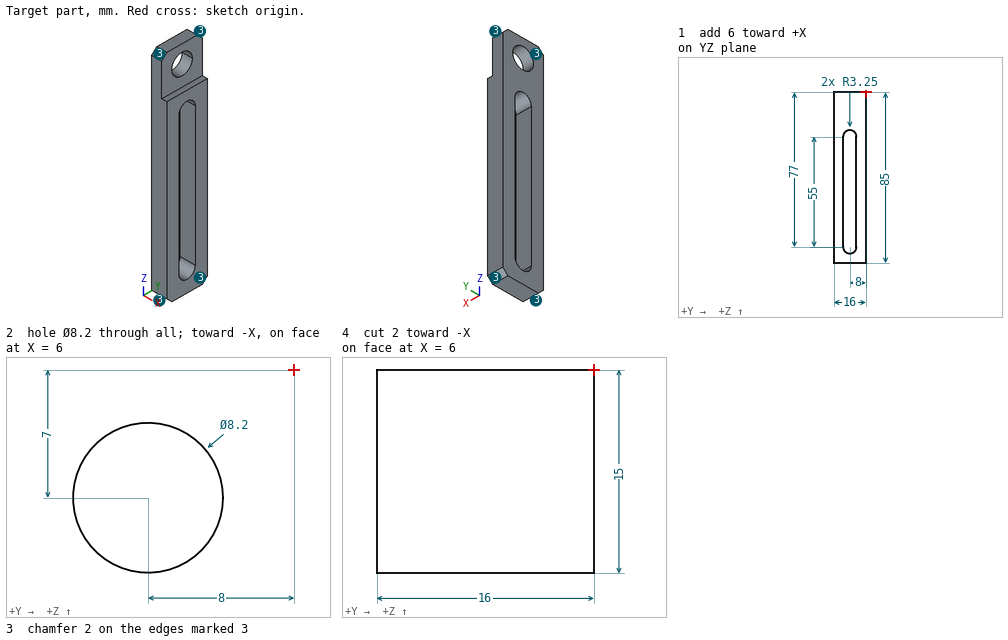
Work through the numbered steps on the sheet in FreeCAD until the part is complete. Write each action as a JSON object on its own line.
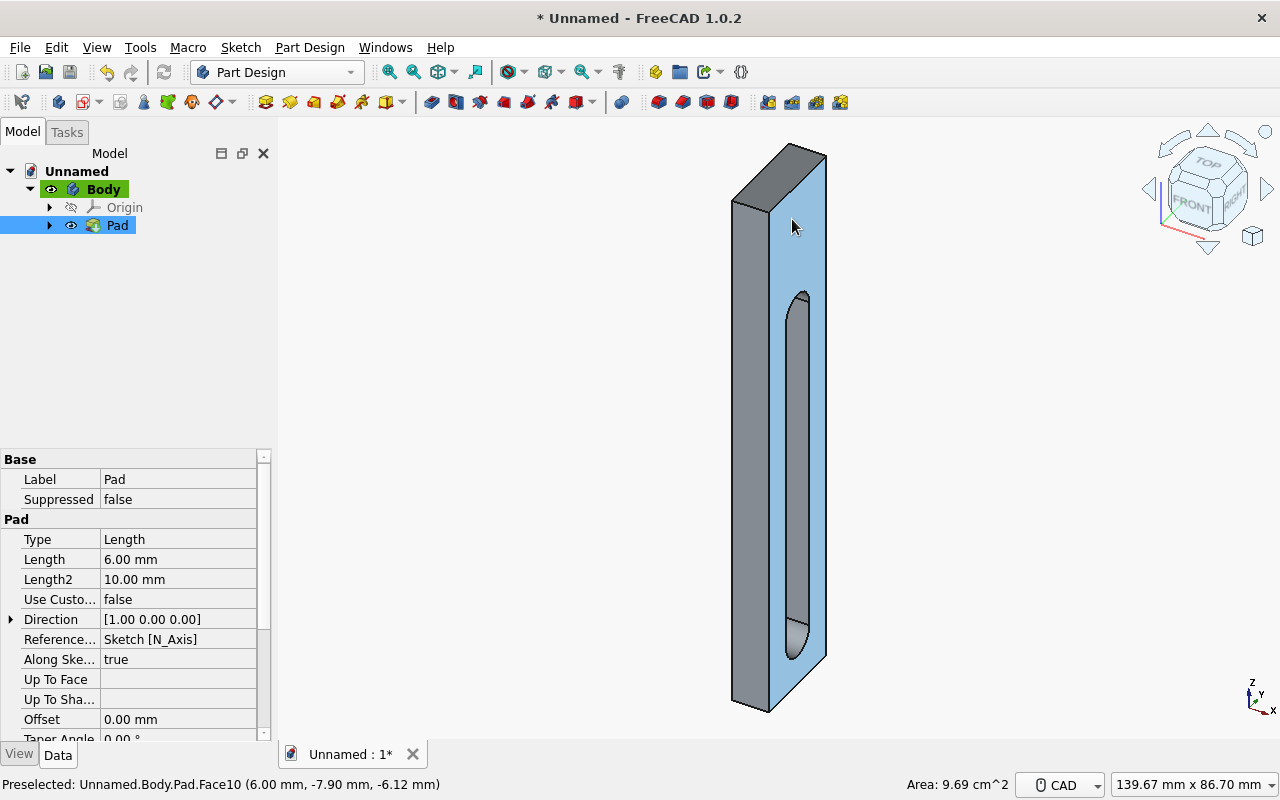
{"action": "left_click", "coordinate": [84, 102]}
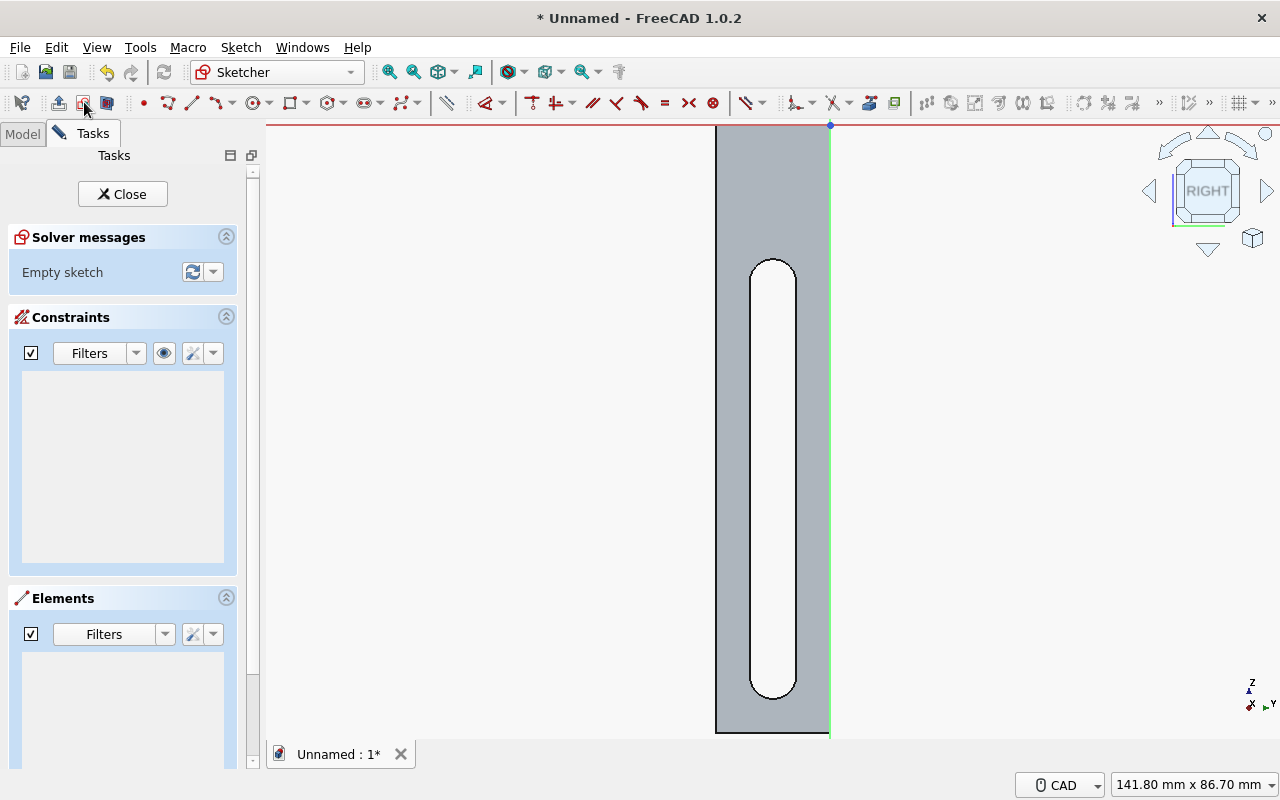
{"action": "scroll", "coordinate": [704, 429], "scroll_direction": "down", "scroll_amount": 5}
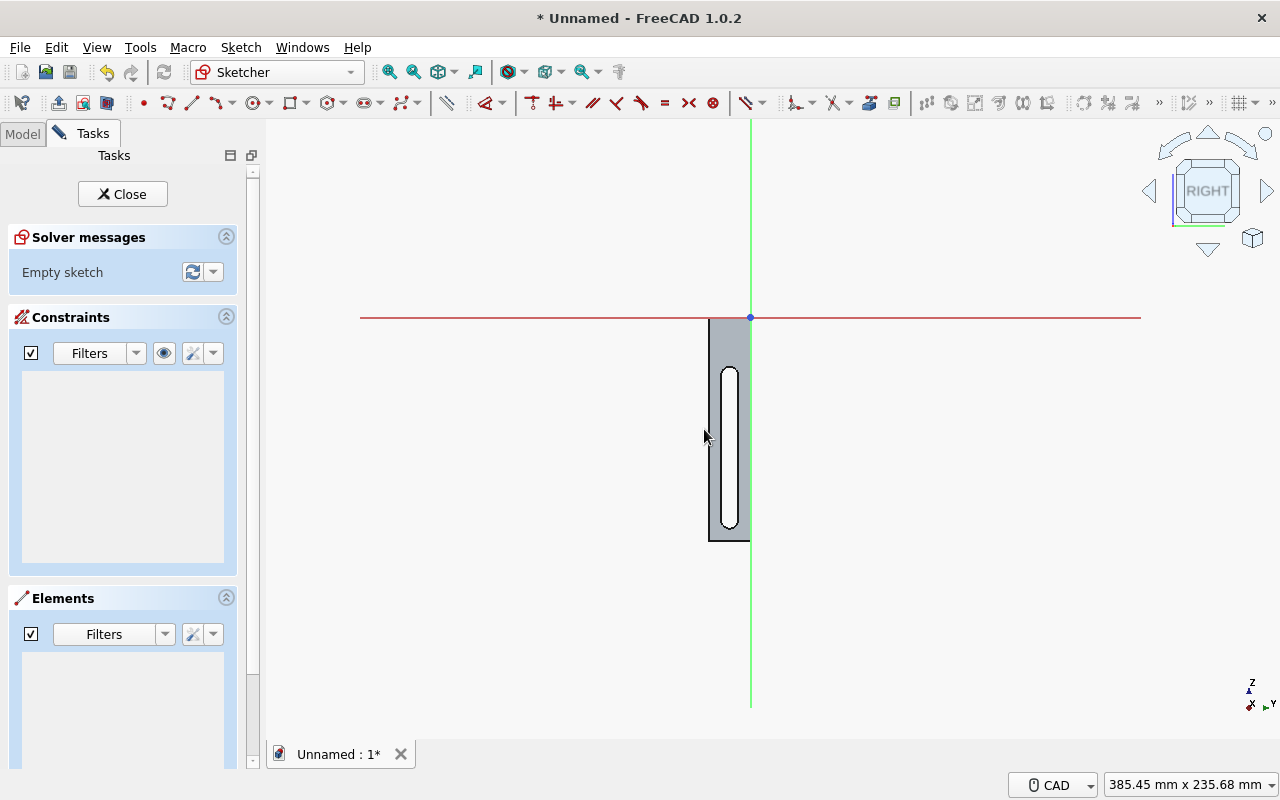
{"action": "scroll", "coordinate": [737, 324], "scroll_direction": "up", "scroll_amount": 13}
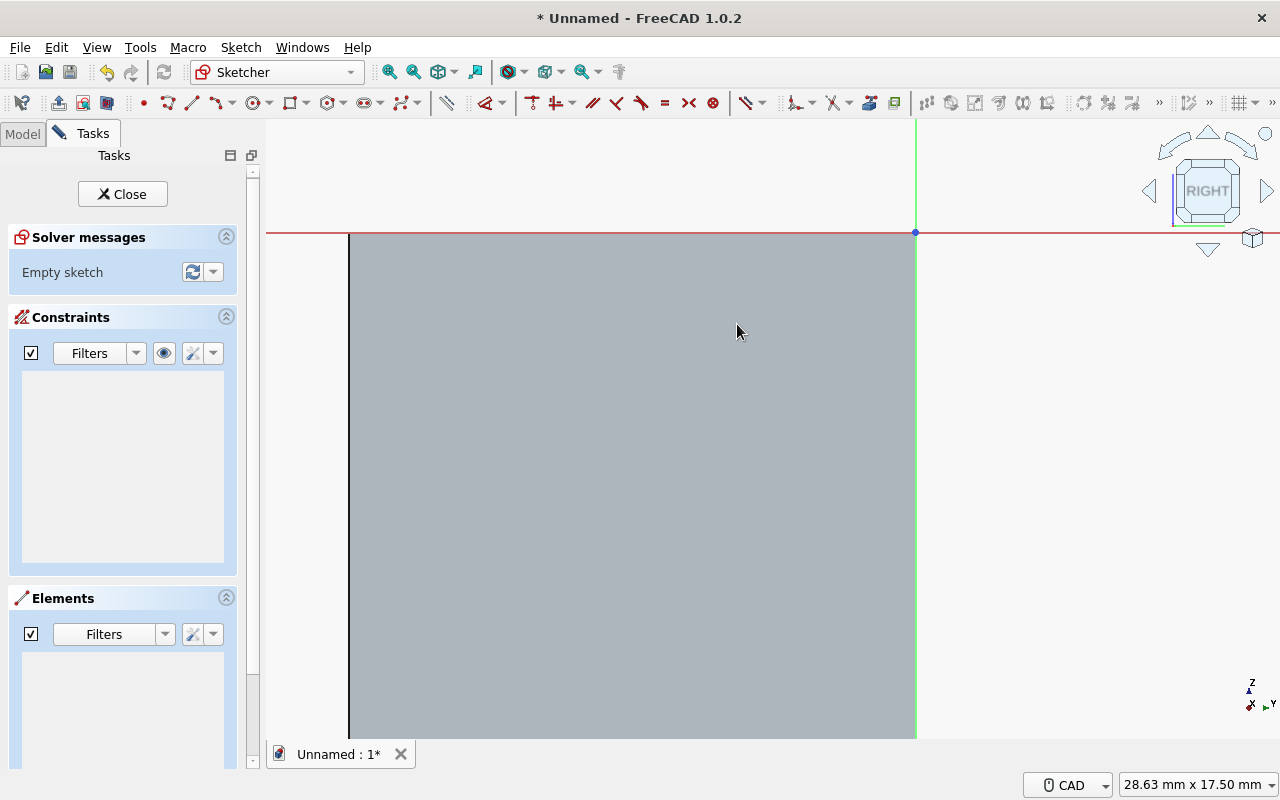
{"action": "key", "text": "g c"}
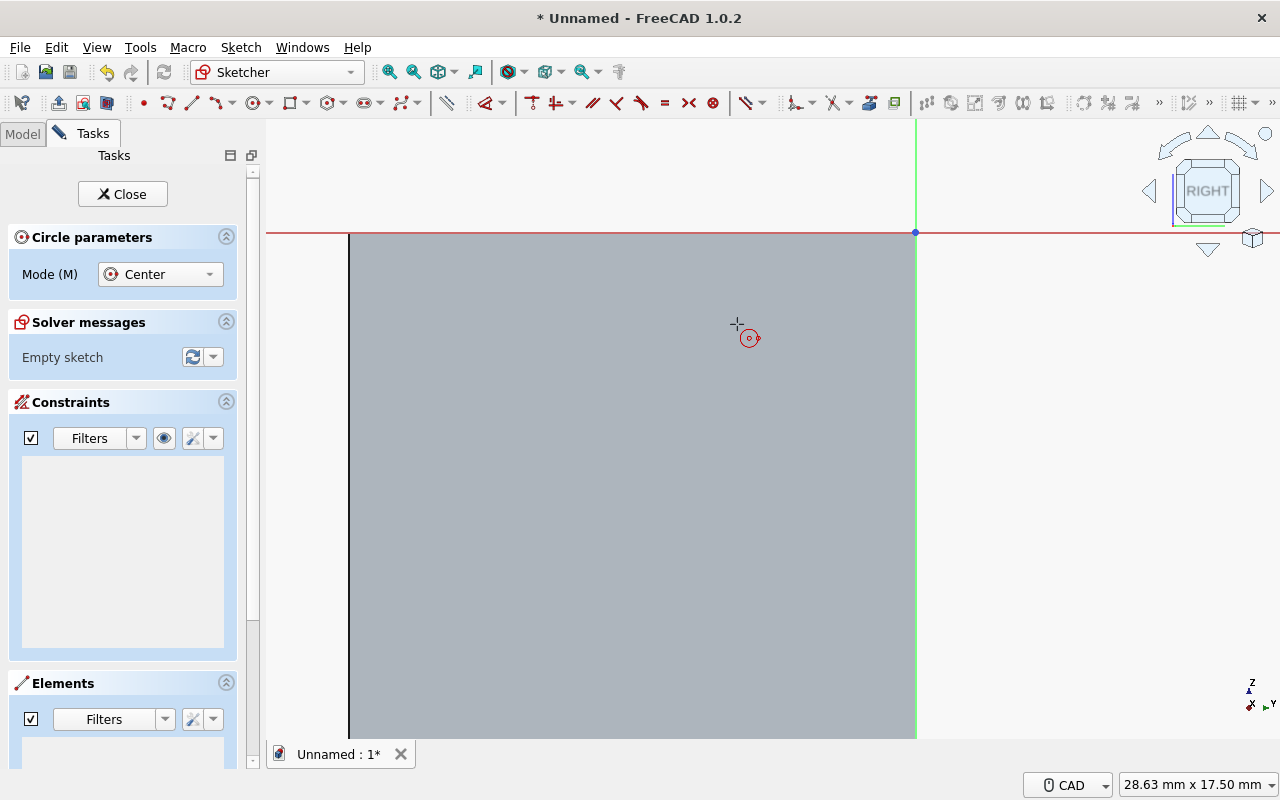
{"action": "left_click", "coordinate": [632, 480]}
{"action": "mouse_move", "coordinate": [735, 378]}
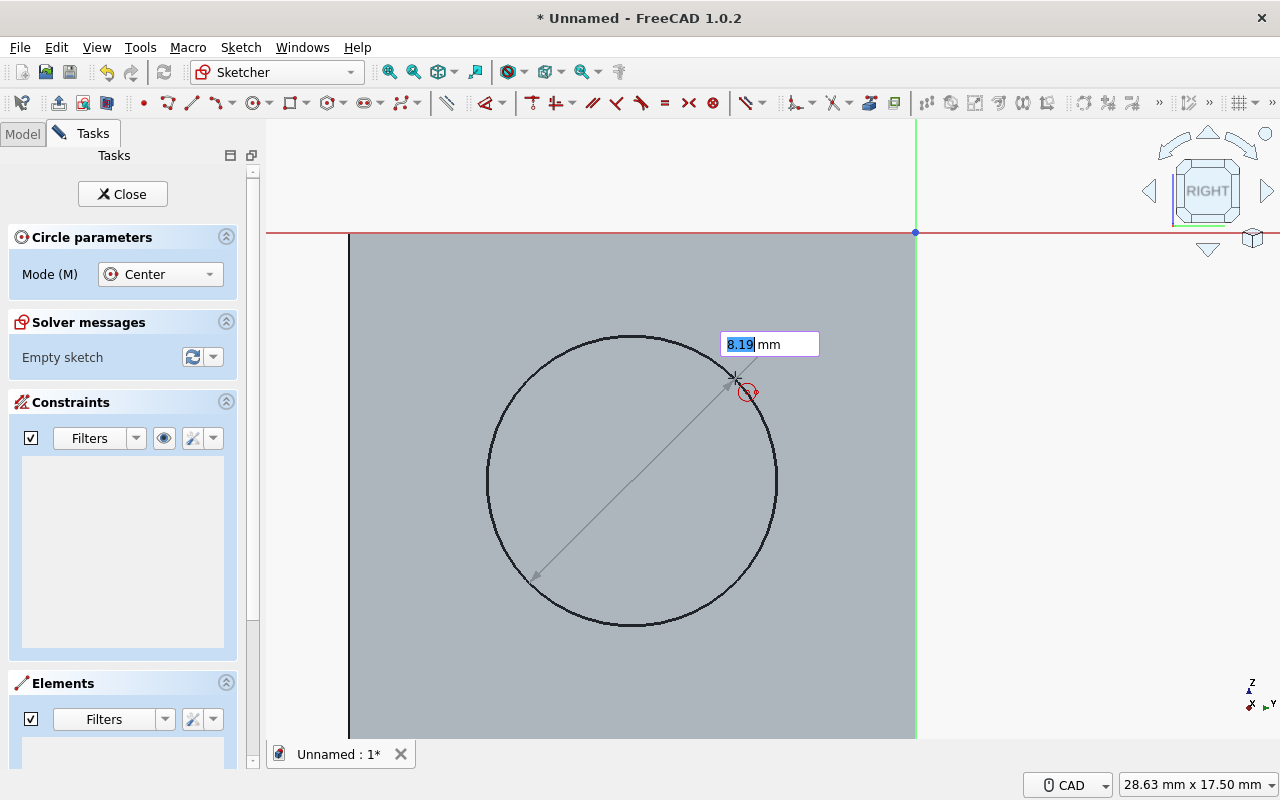
{"action": "type", "text": "8.2"}
{"action": "key", "text": "Return"}
{"action": "key", "text": "Escape"}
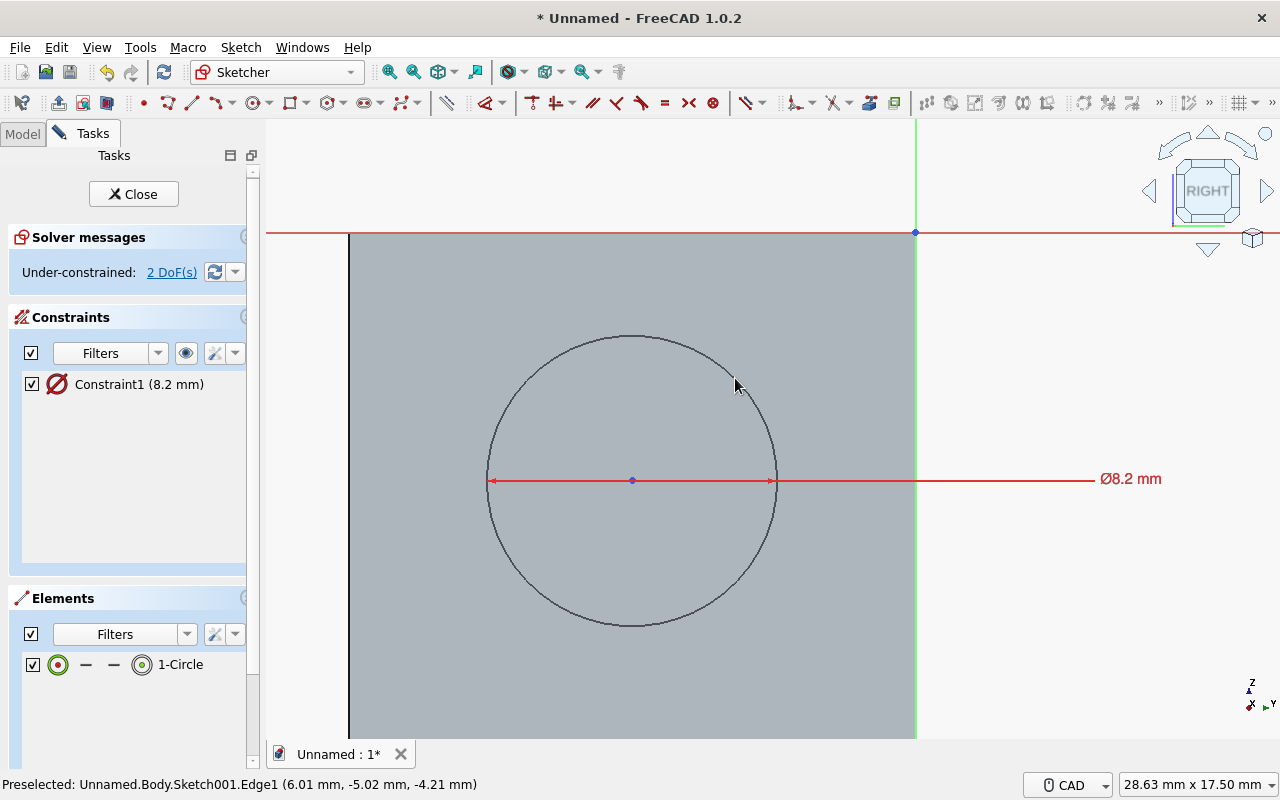
{"action": "left_click", "coordinate": [486, 104]}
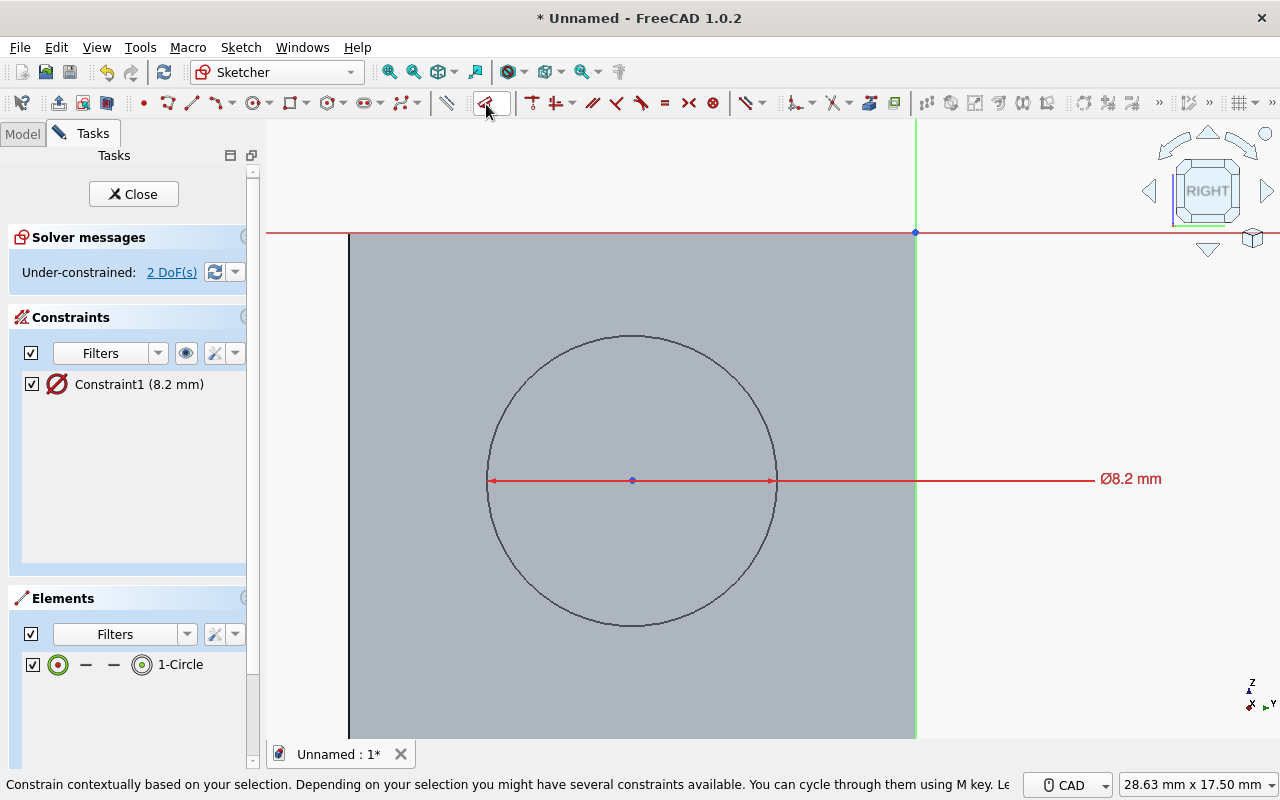
{"action": "left_click", "coordinate": [632, 481]}
{"action": "left_click", "coordinate": [774, 199]}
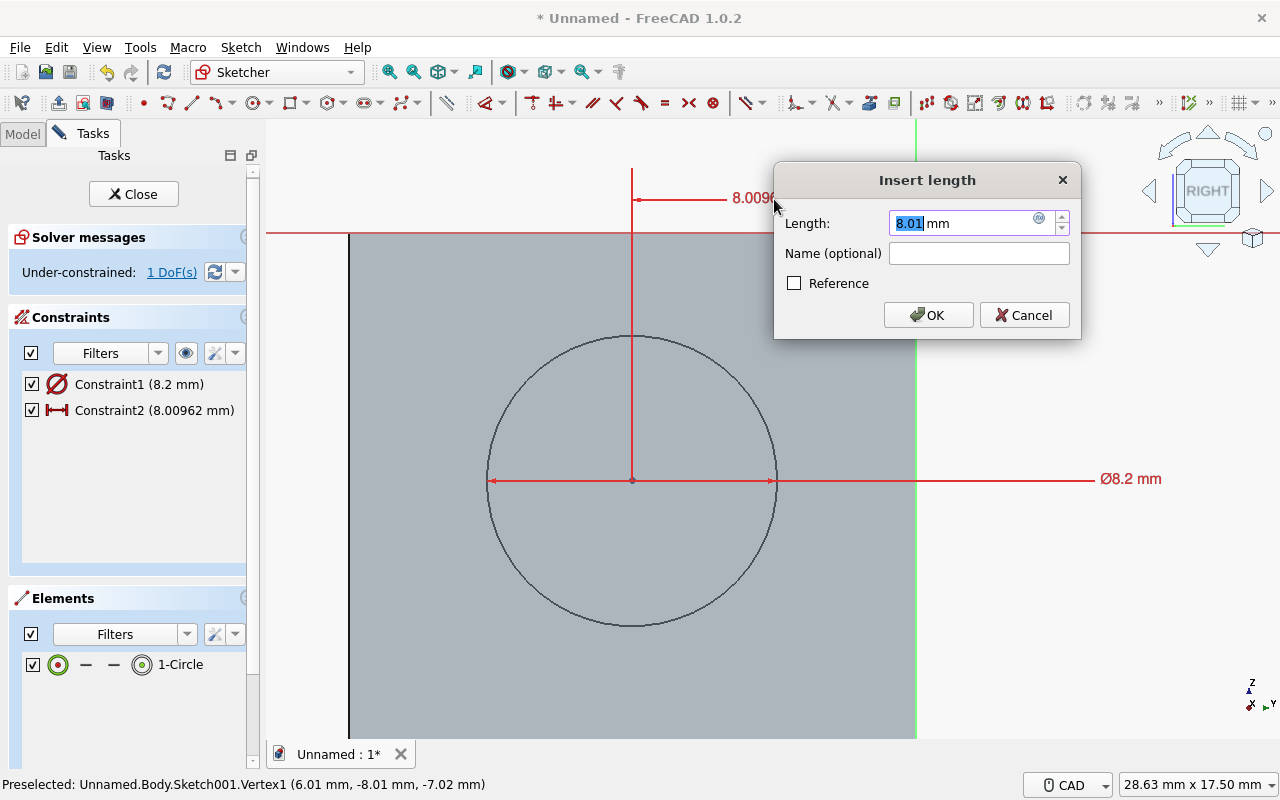
{"action": "type", "text": "8"}
{"action": "key", "text": "Return"}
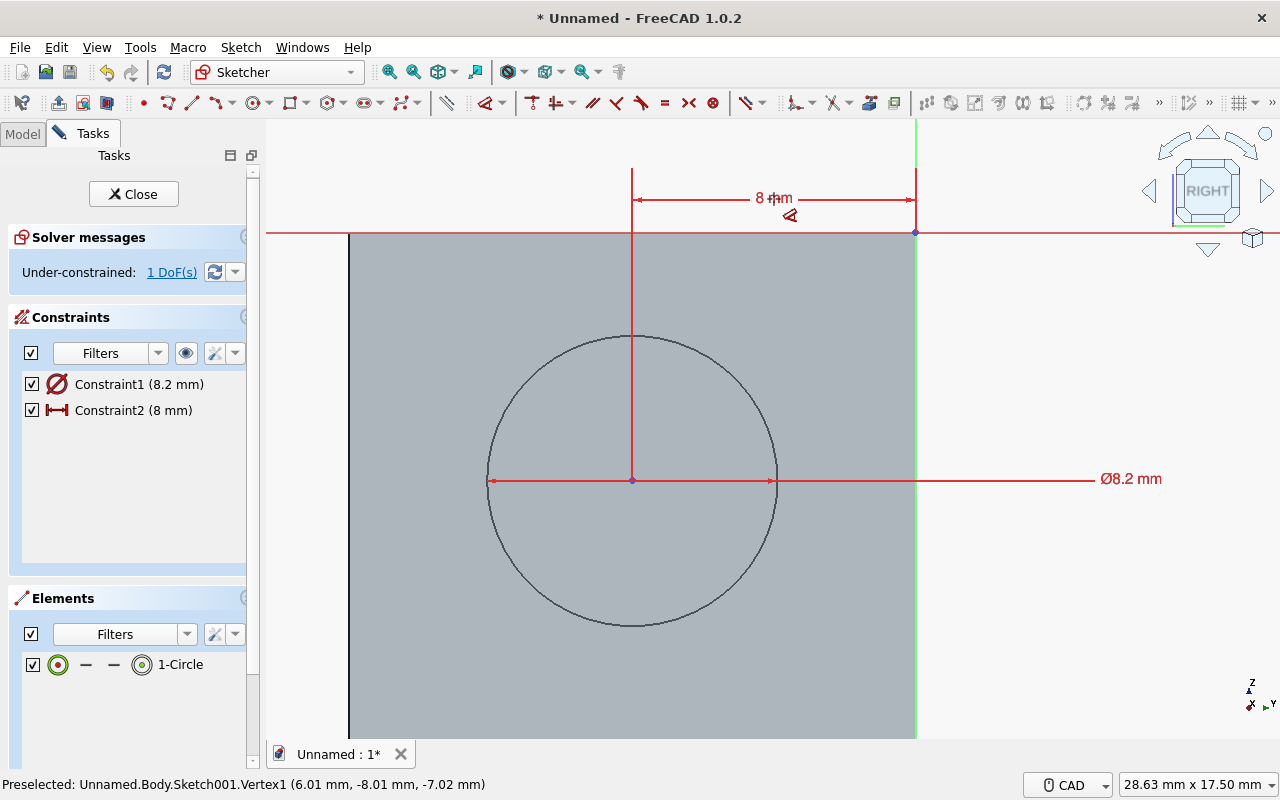
{"action": "left_click", "coordinate": [632, 481]}
{"action": "left_click", "coordinate": [950, 357]}